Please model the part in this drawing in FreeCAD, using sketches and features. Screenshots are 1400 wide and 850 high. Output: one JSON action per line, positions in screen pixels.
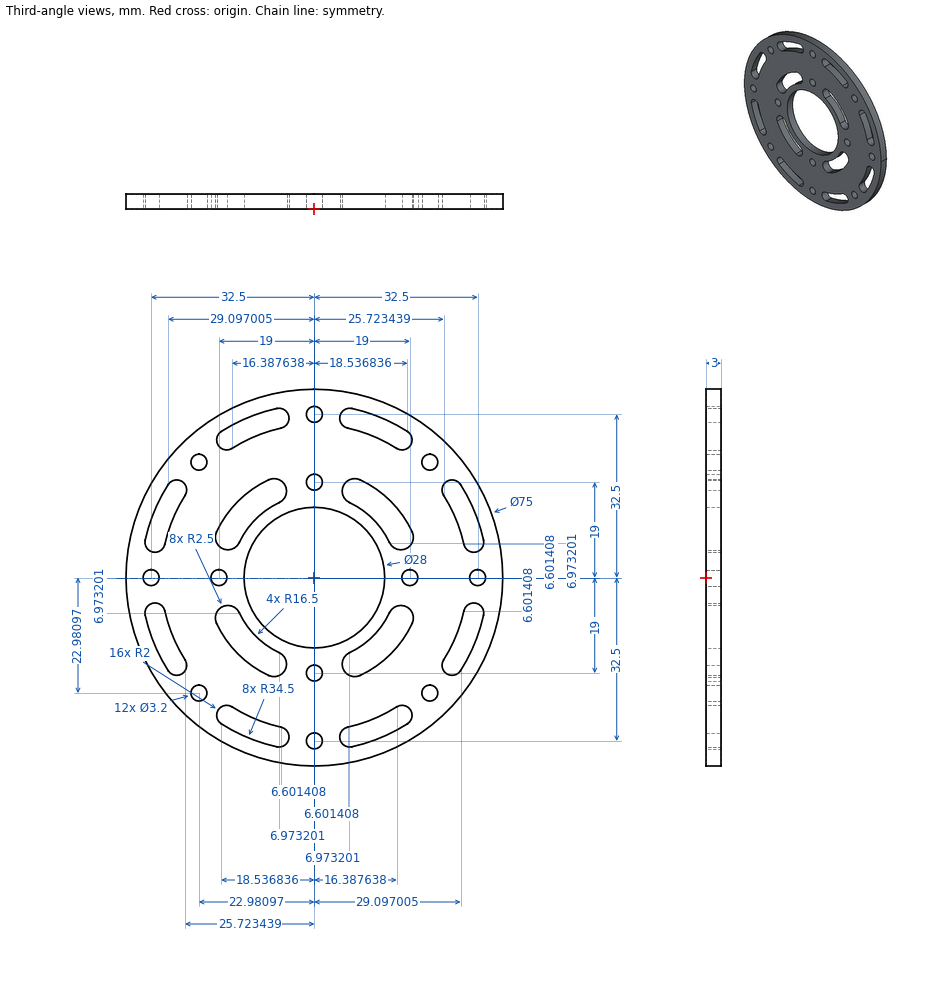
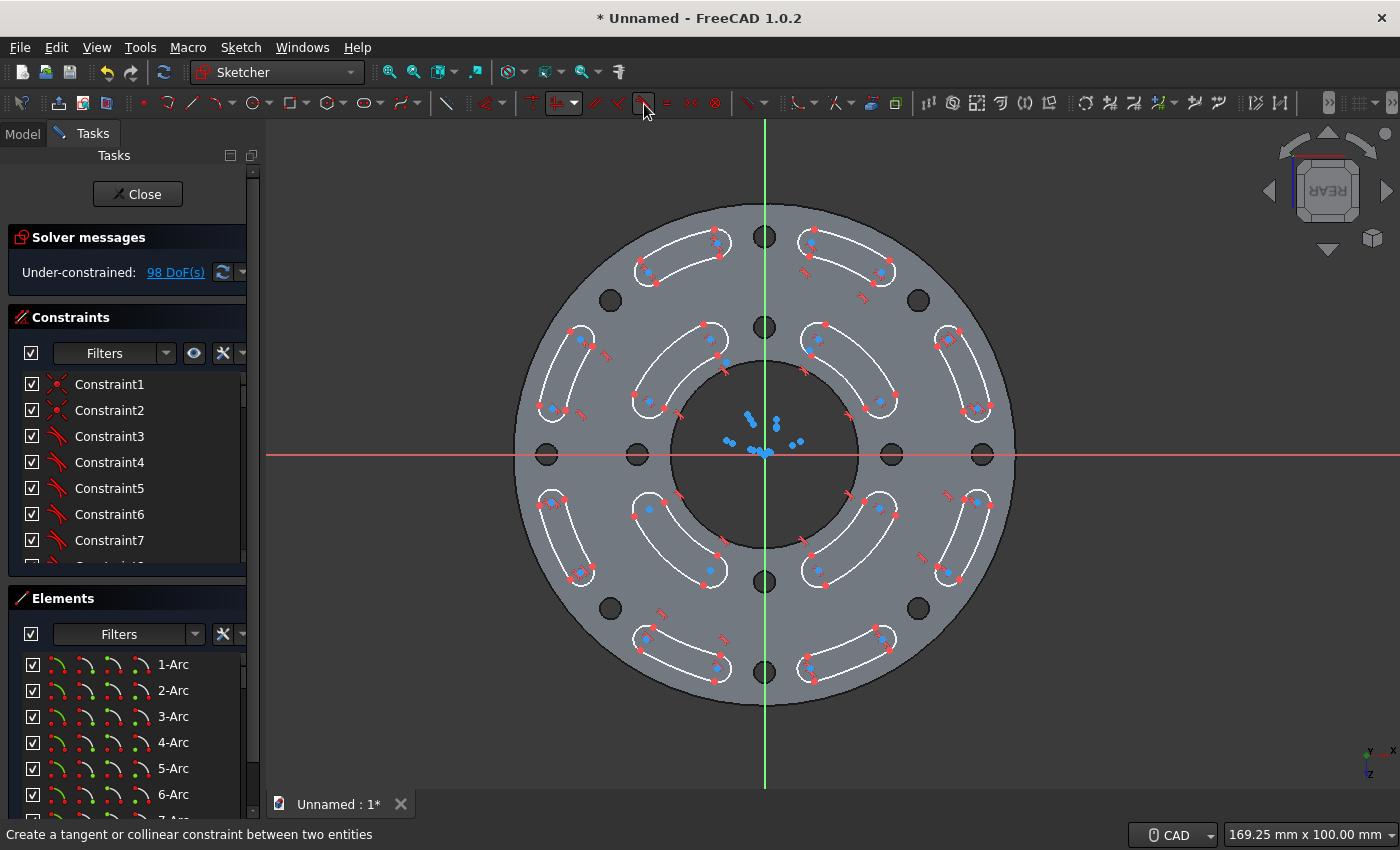
{"action": "left_click", "coordinate": [652, 493]}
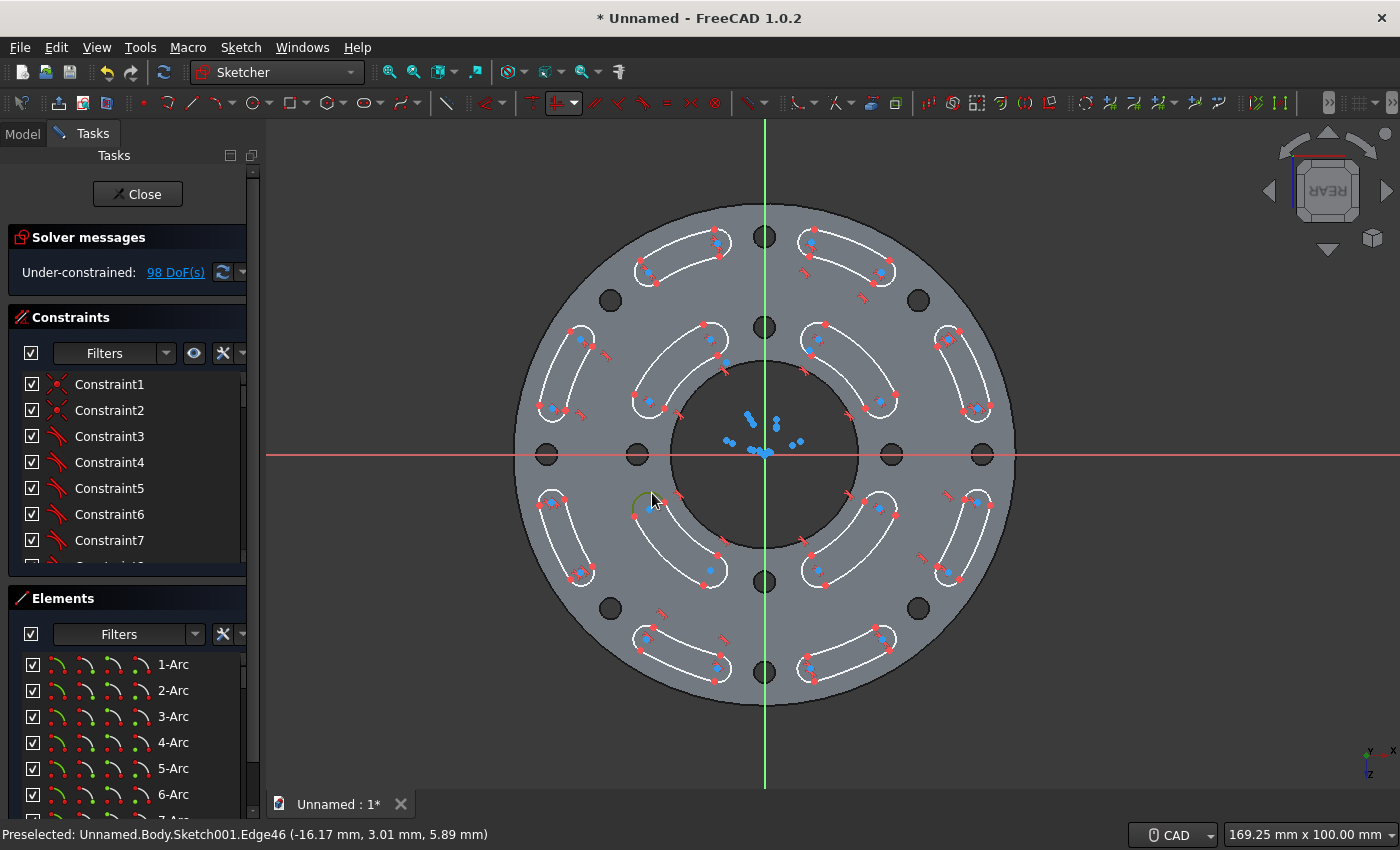
{"action": "left_click", "coordinate": [650, 542]}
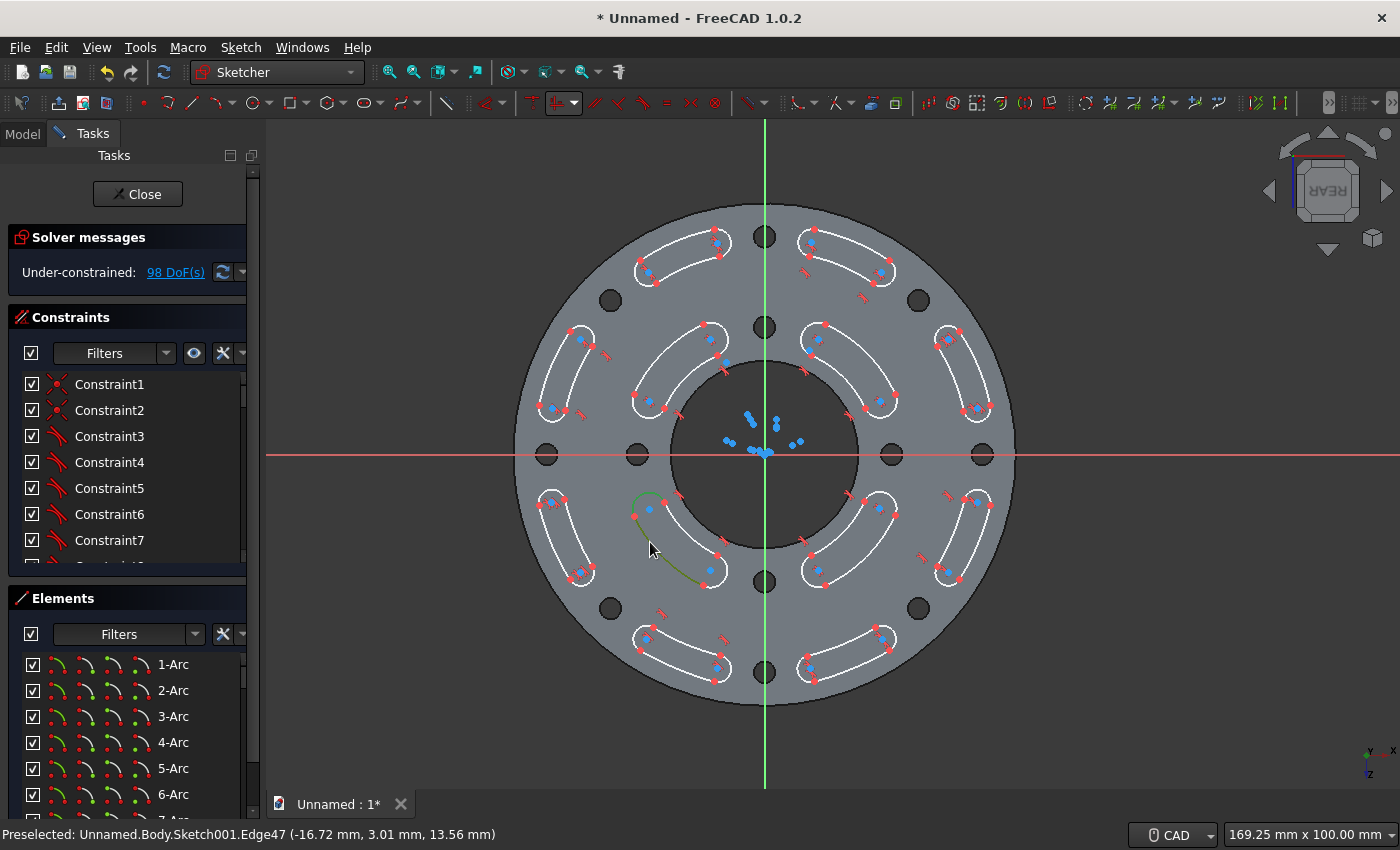
{"action": "left_click", "coordinate": [644, 104]}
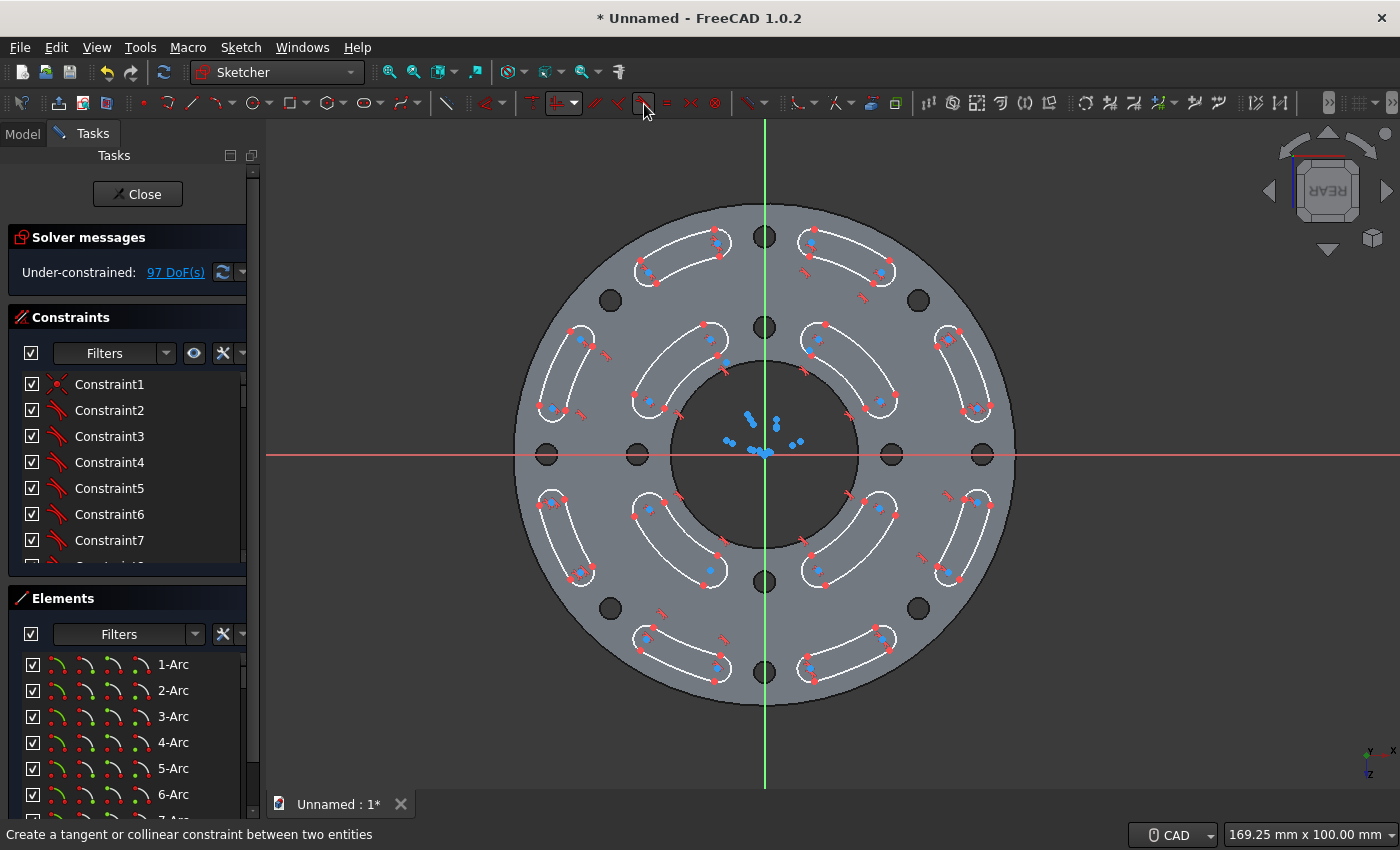
{"action": "left_click", "coordinate": [650, 542]}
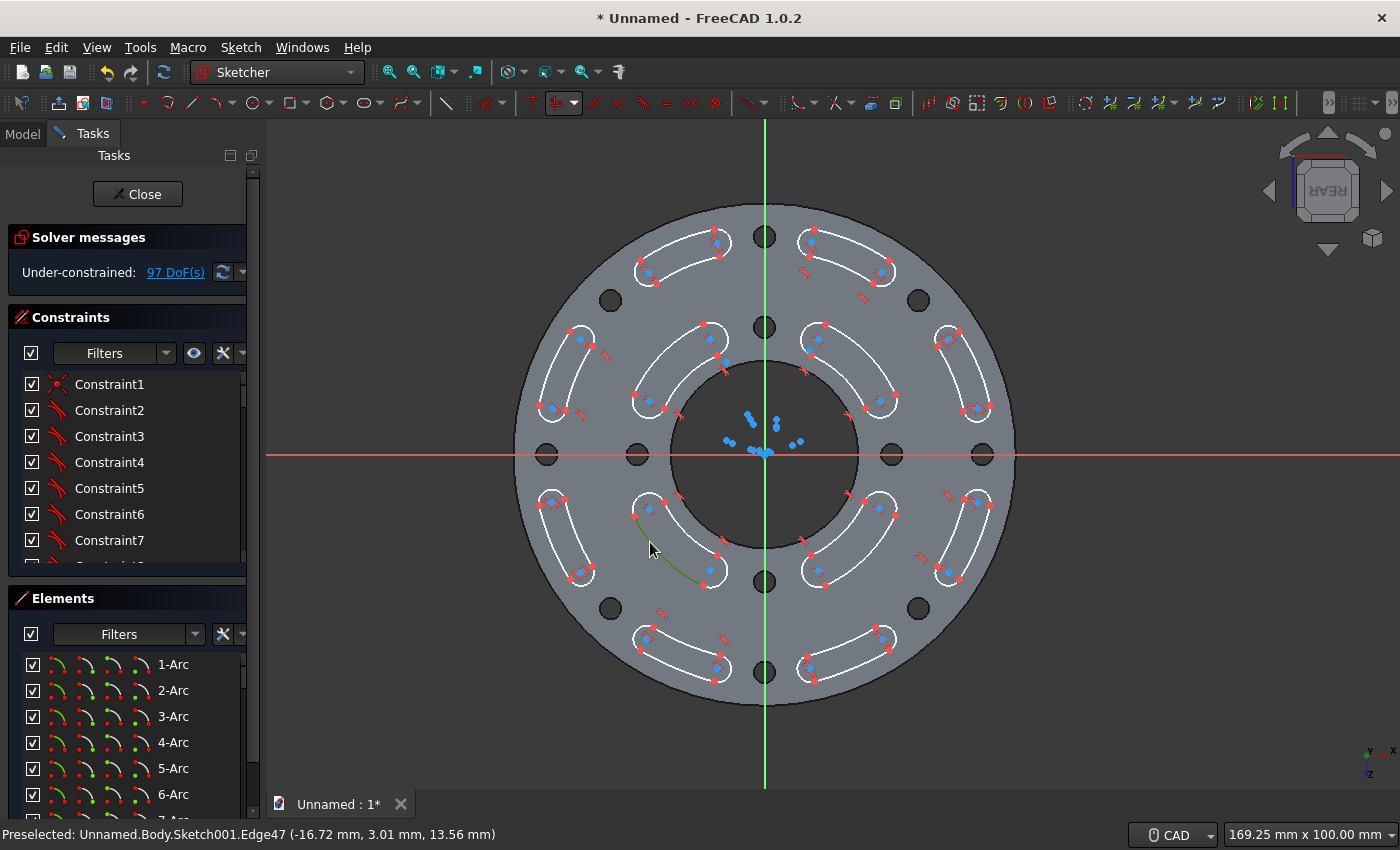
{"action": "left_click", "coordinate": [719, 585]}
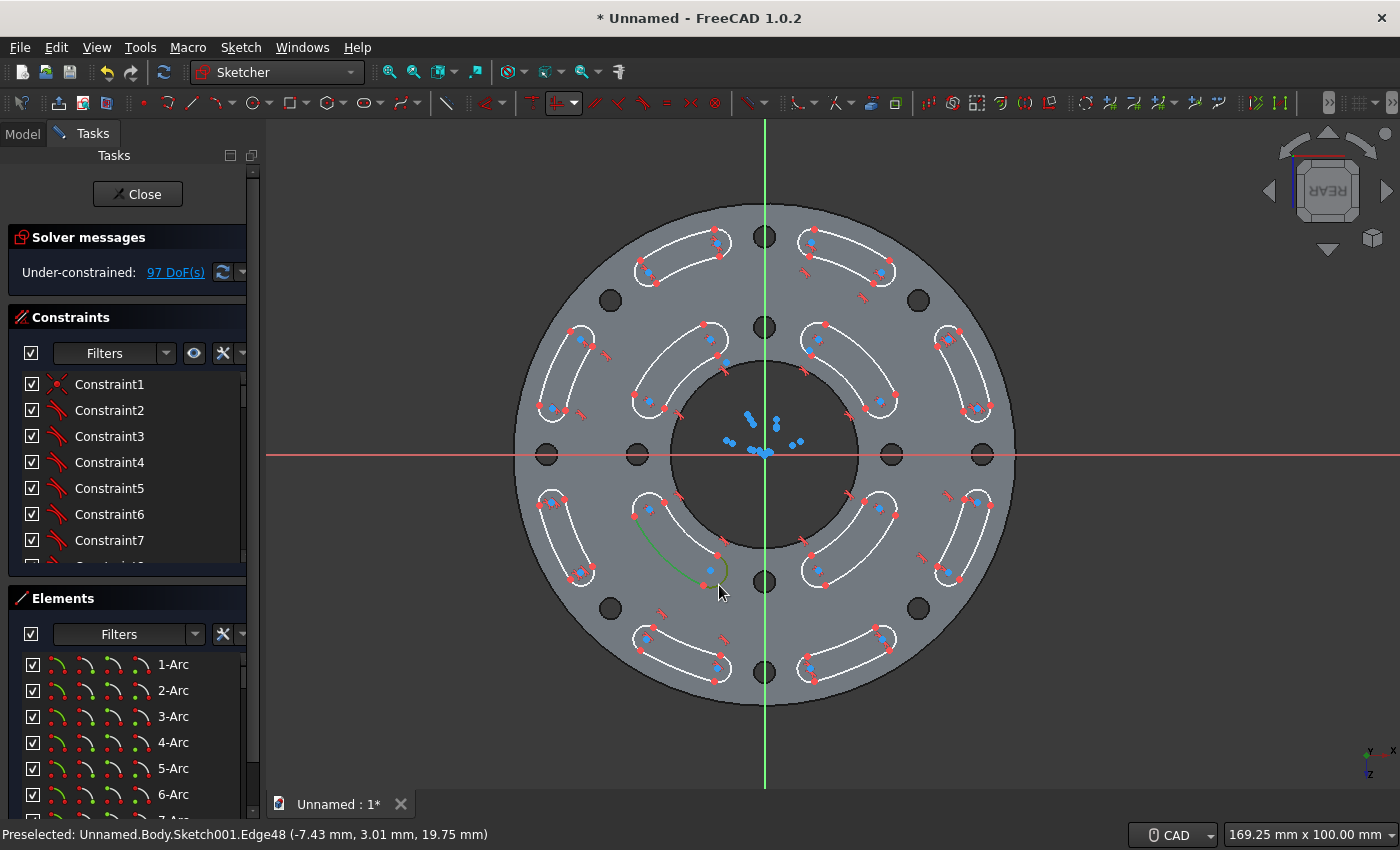
{"action": "left_click", "coordinate": [644, 104]}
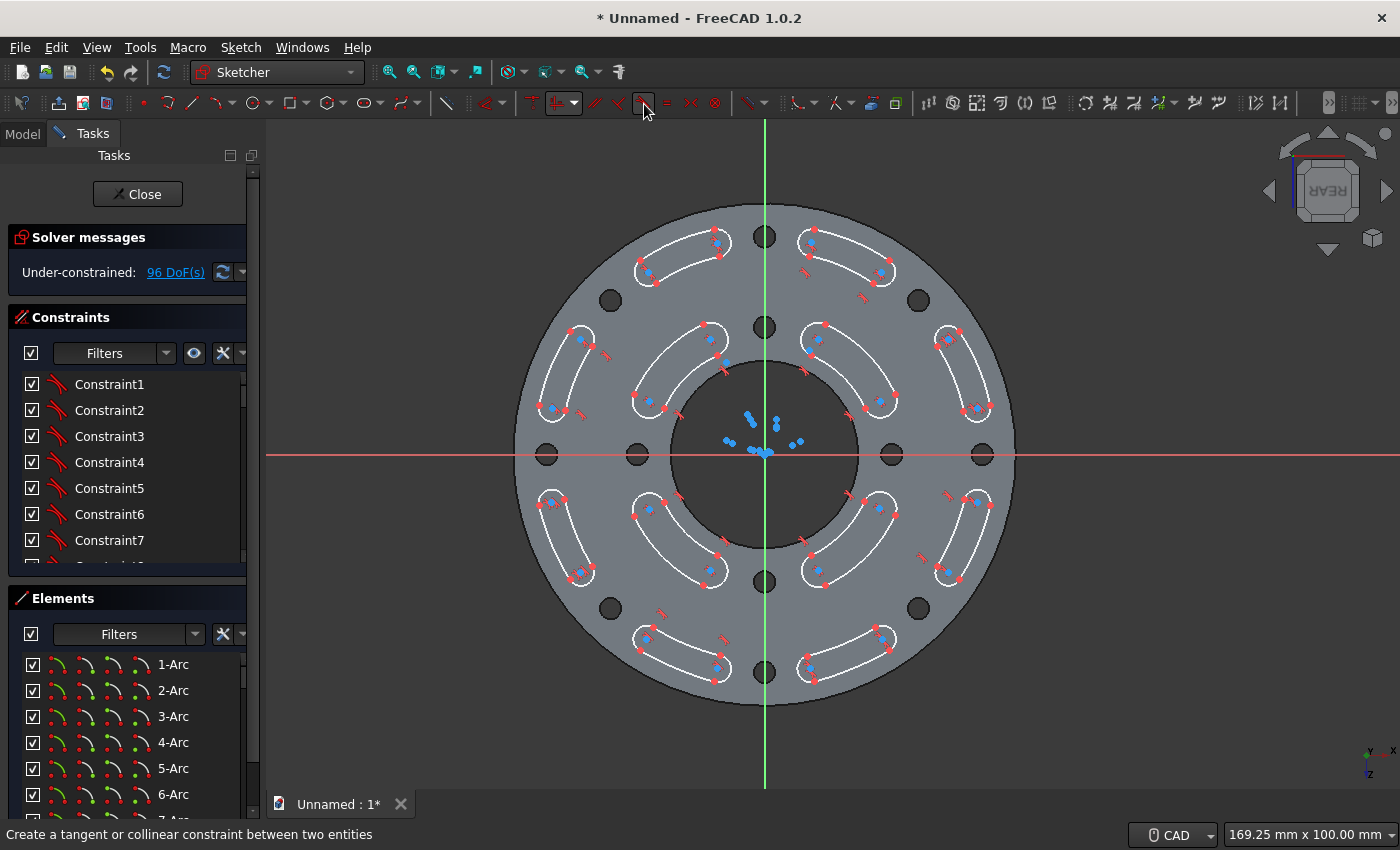
{"action": "left_click", "coordinate": [691, 236]}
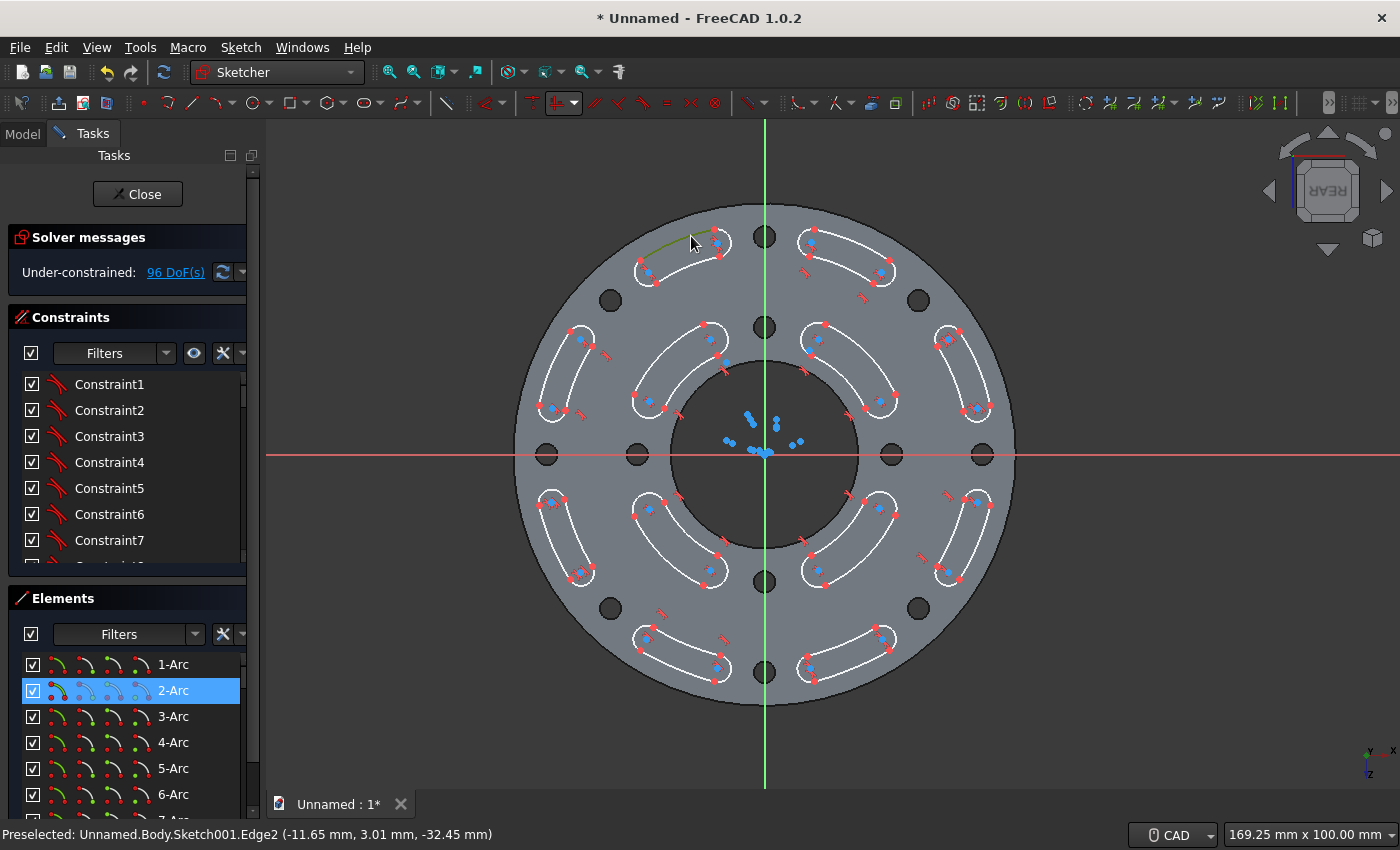
{"action": "left_click", "coordinate": [700, 262]}